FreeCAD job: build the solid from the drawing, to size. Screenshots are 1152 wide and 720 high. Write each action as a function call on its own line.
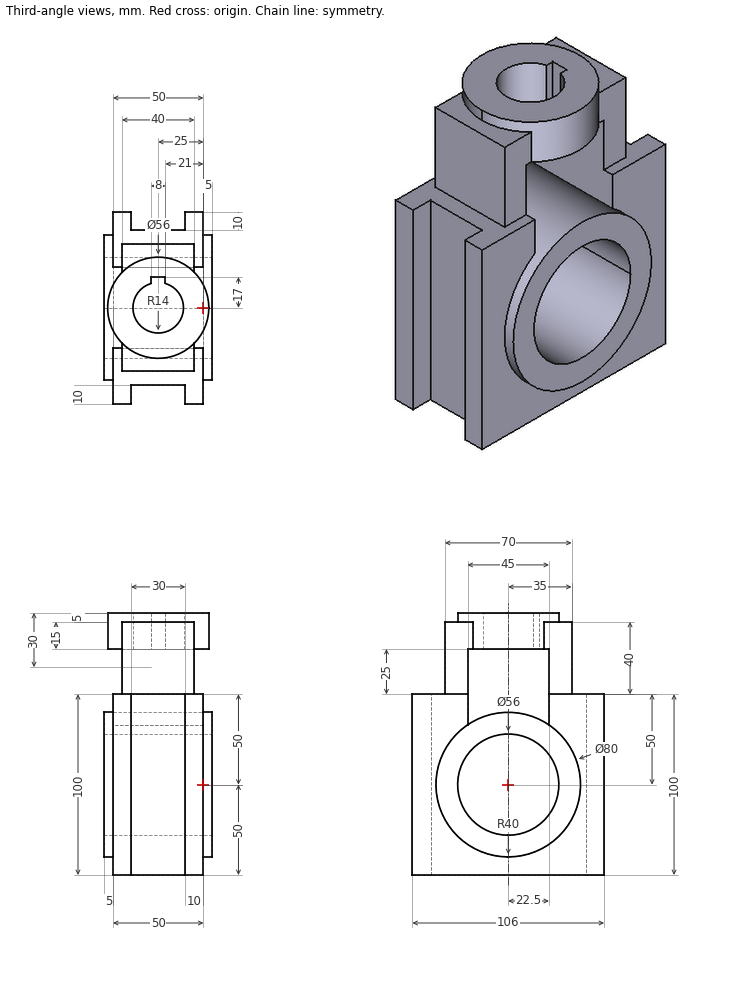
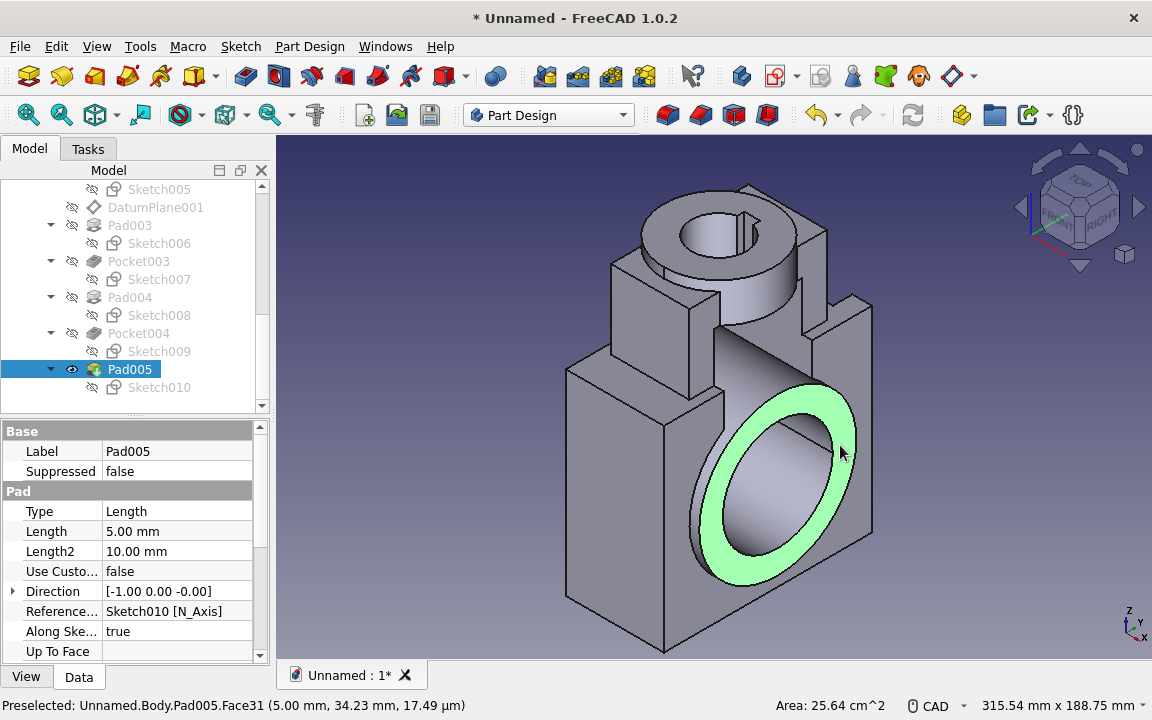
click(774, 76)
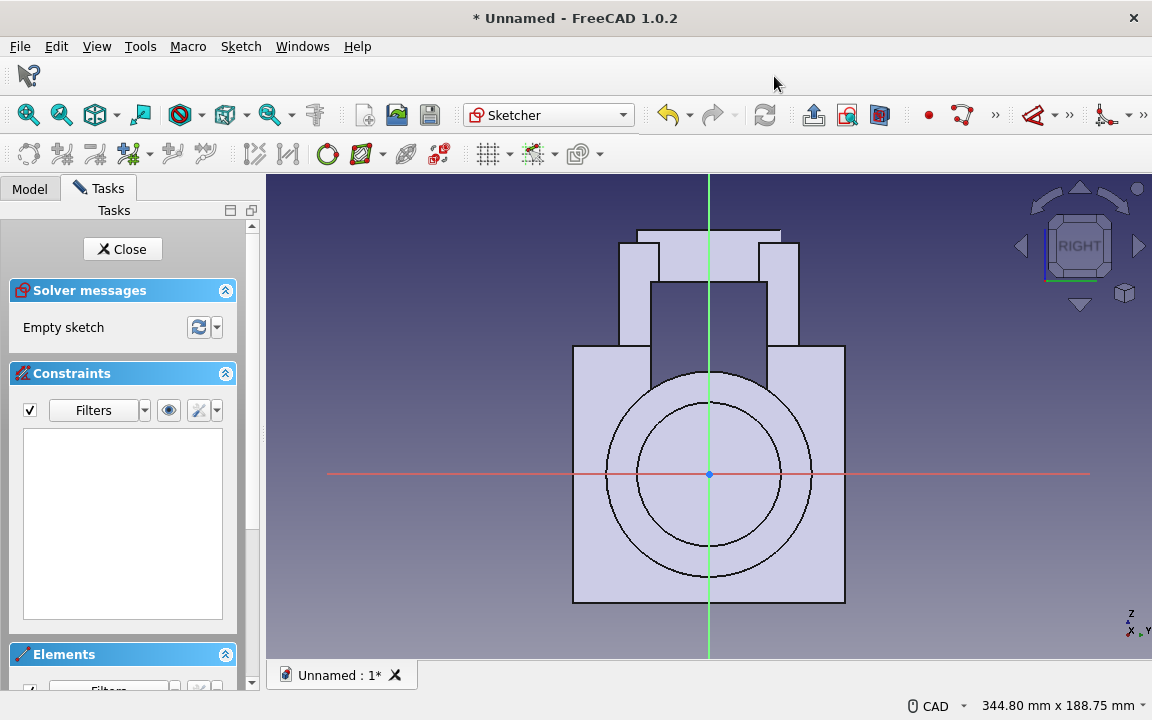
scroll(765, 521, up, 4)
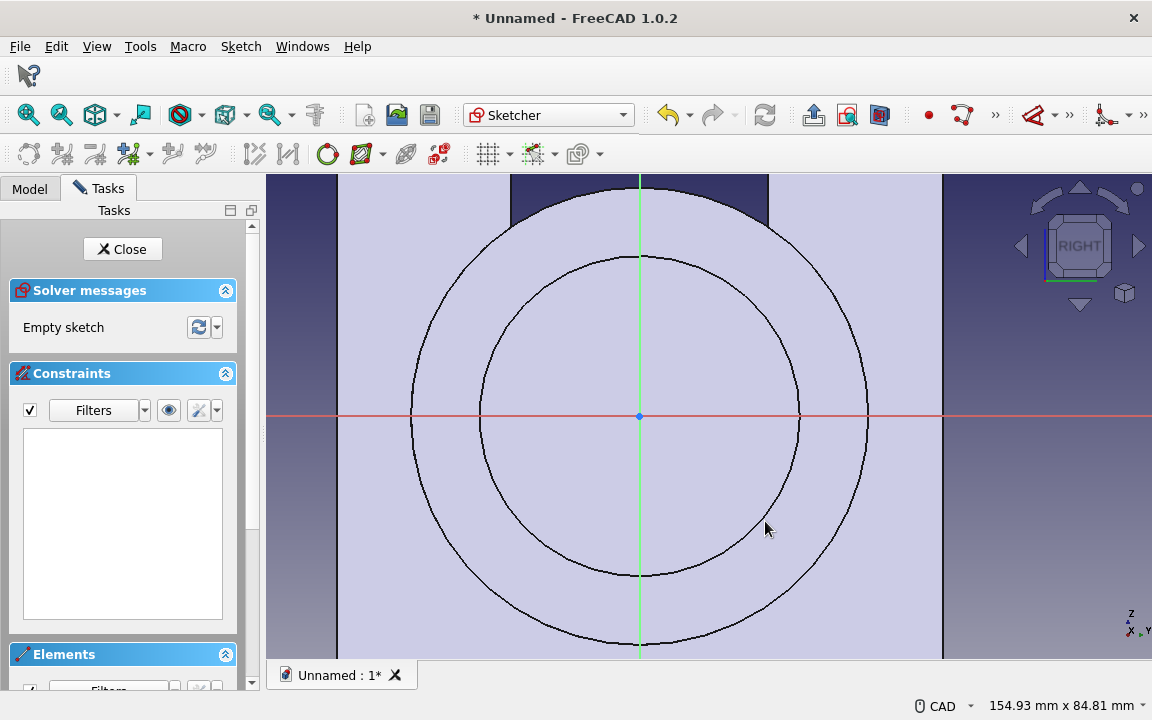
key(g)
key(c)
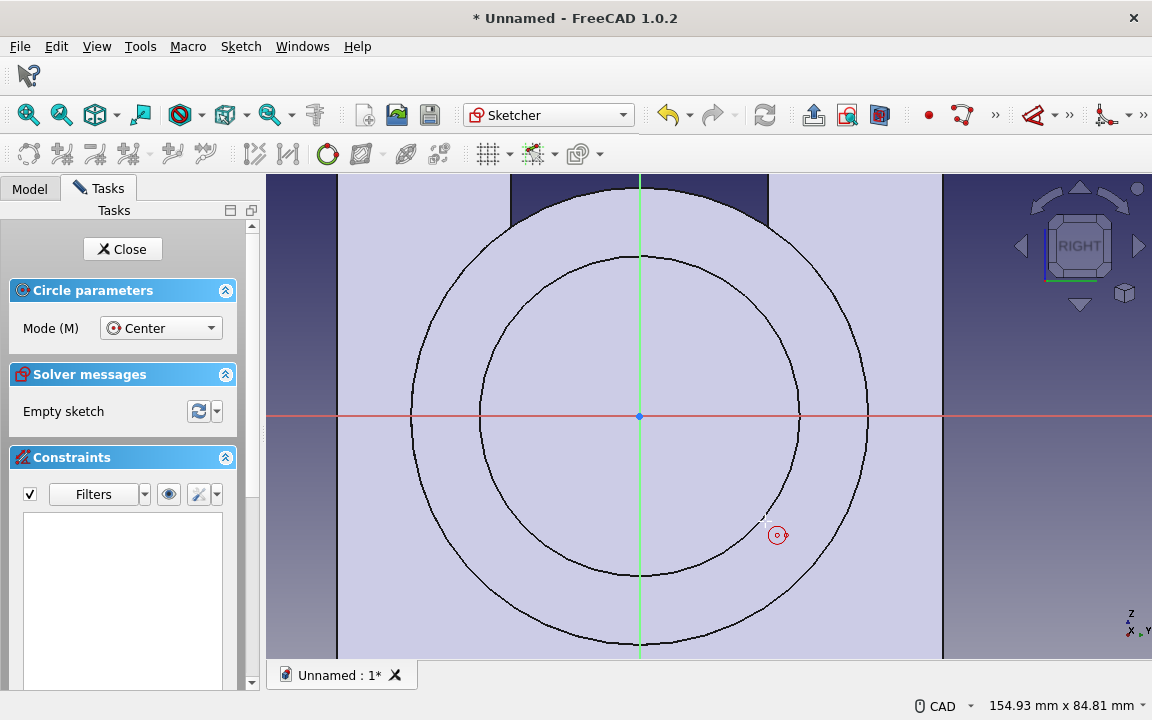
click(640, 416)
move(753, 303)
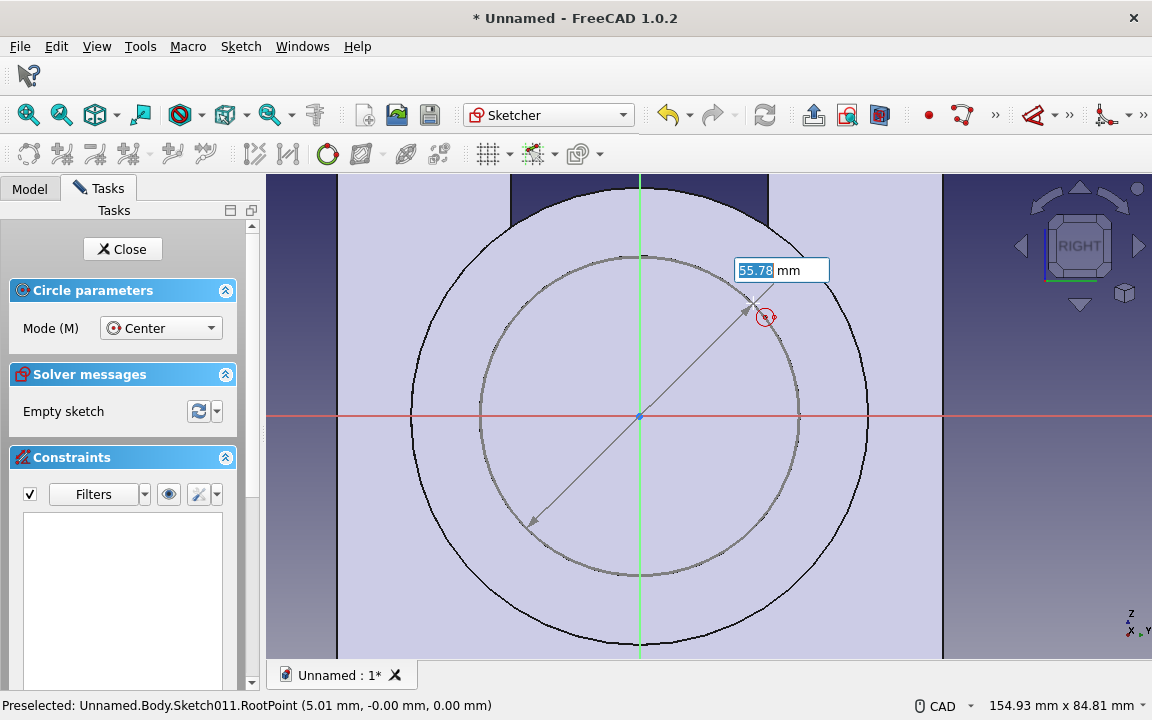
text(56)
key(Return)
key(Escape)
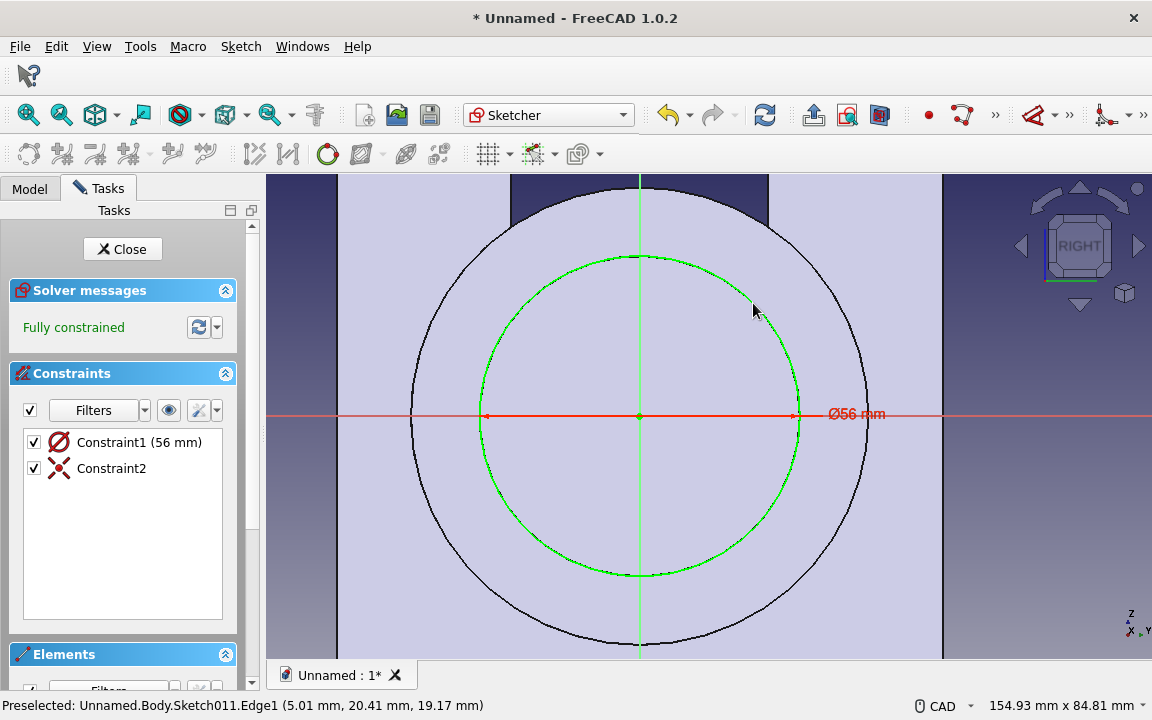
click(123, 249)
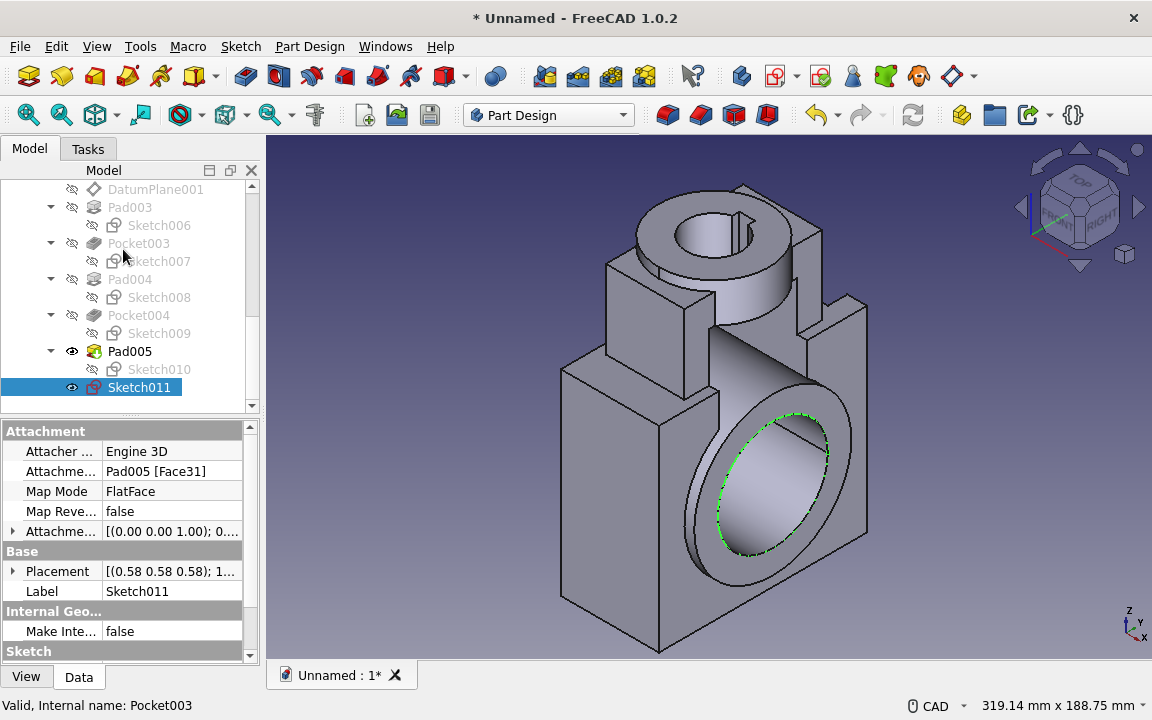
click(246, 76)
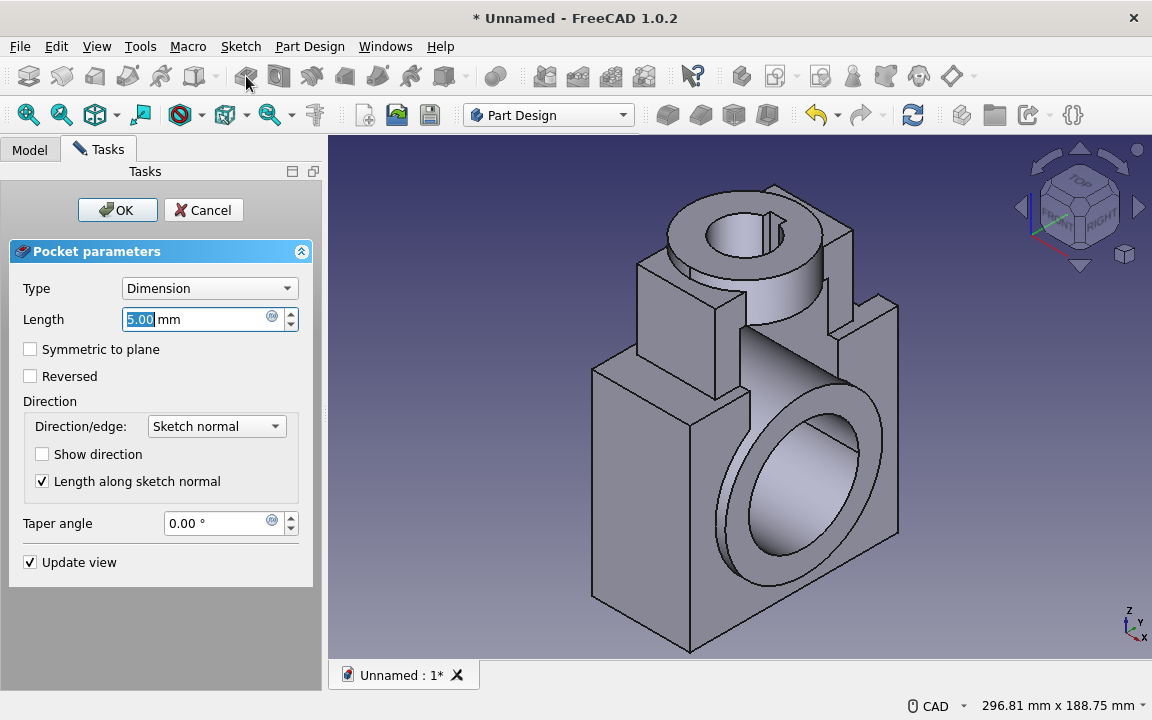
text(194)
key(Tab)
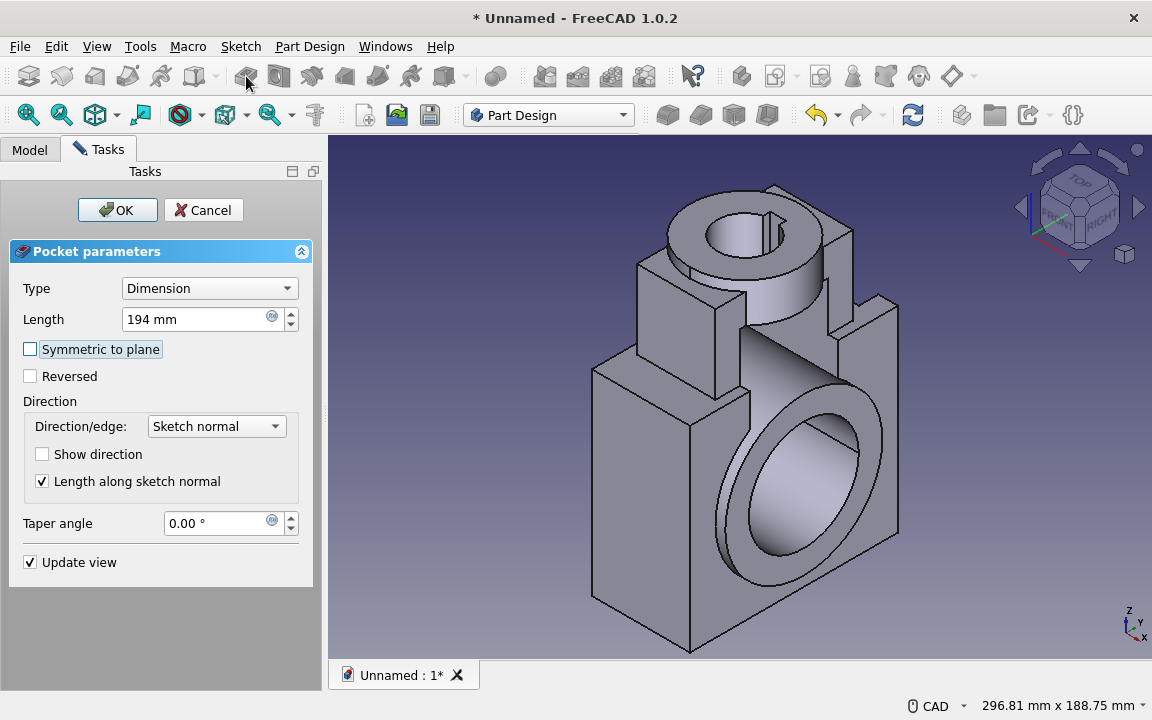
click(118, 210)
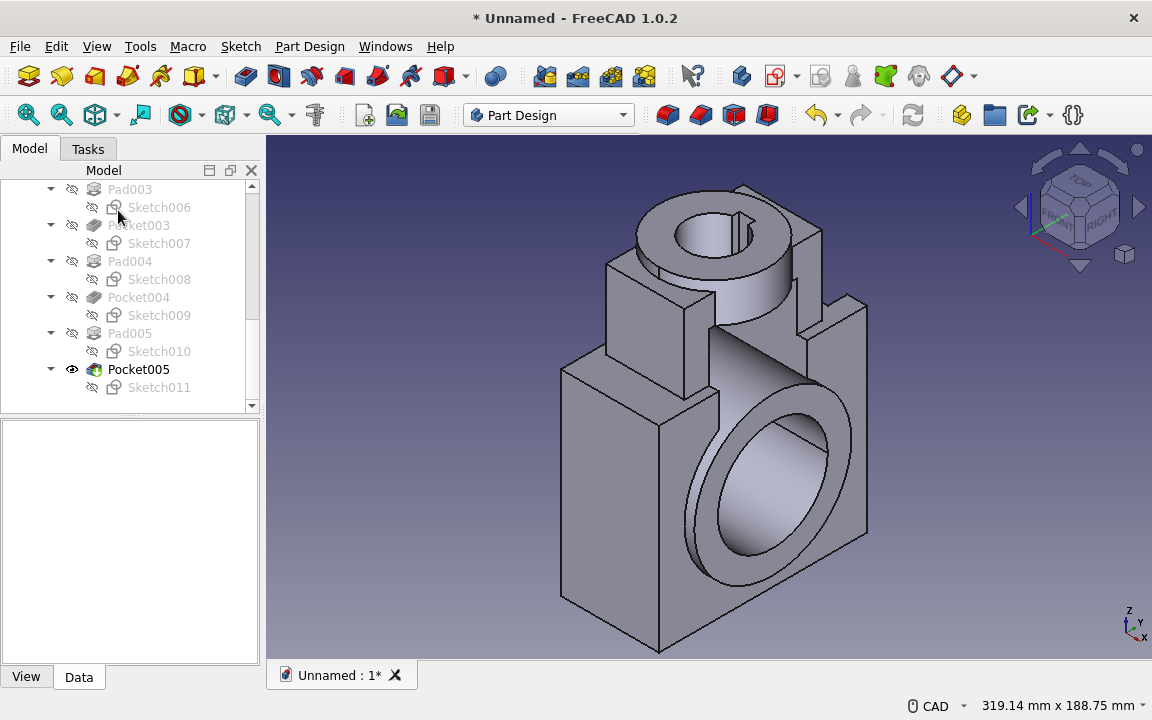
click(610, 542)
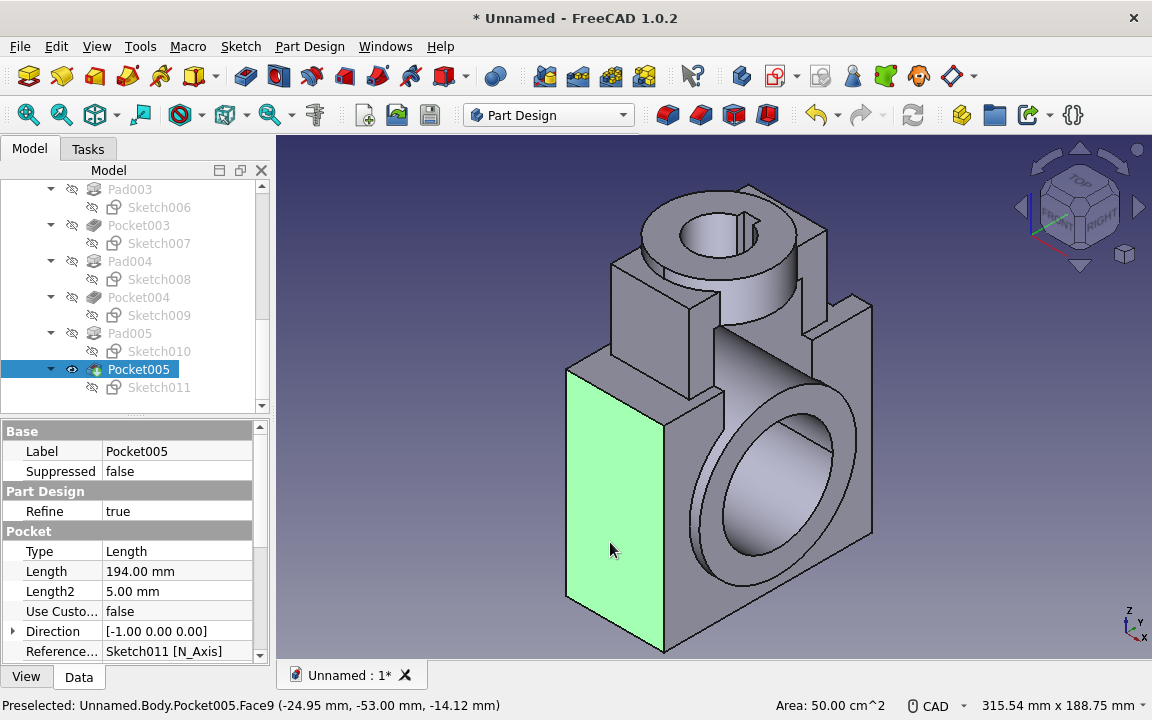
click(774, 76)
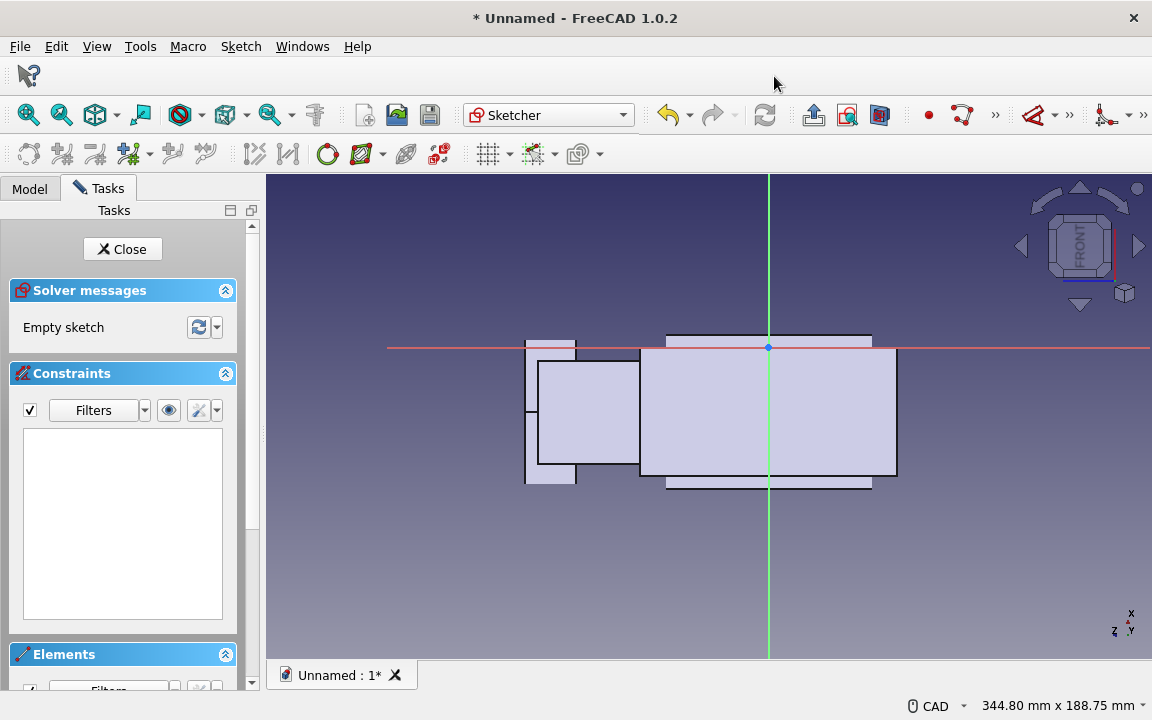
scroll(925, 378, up, 3)